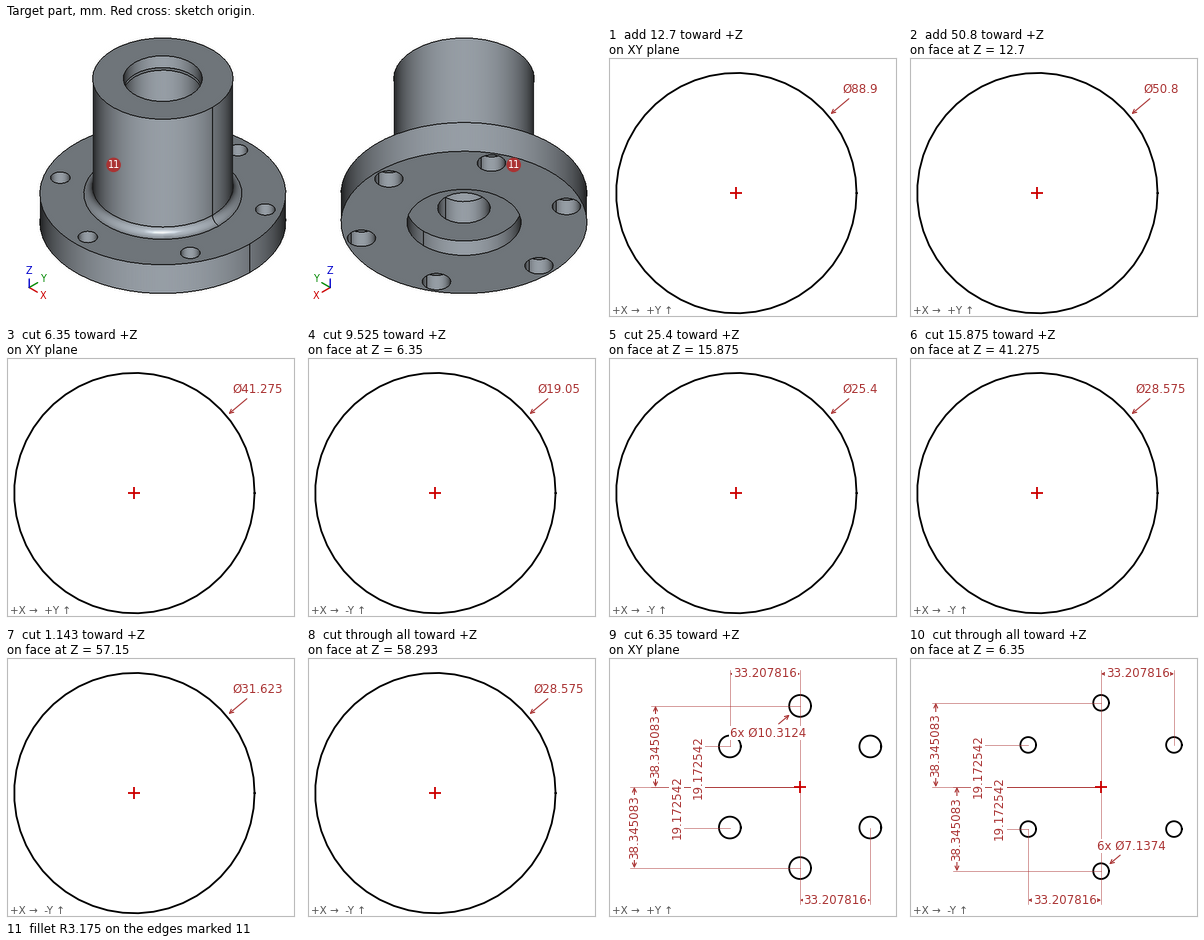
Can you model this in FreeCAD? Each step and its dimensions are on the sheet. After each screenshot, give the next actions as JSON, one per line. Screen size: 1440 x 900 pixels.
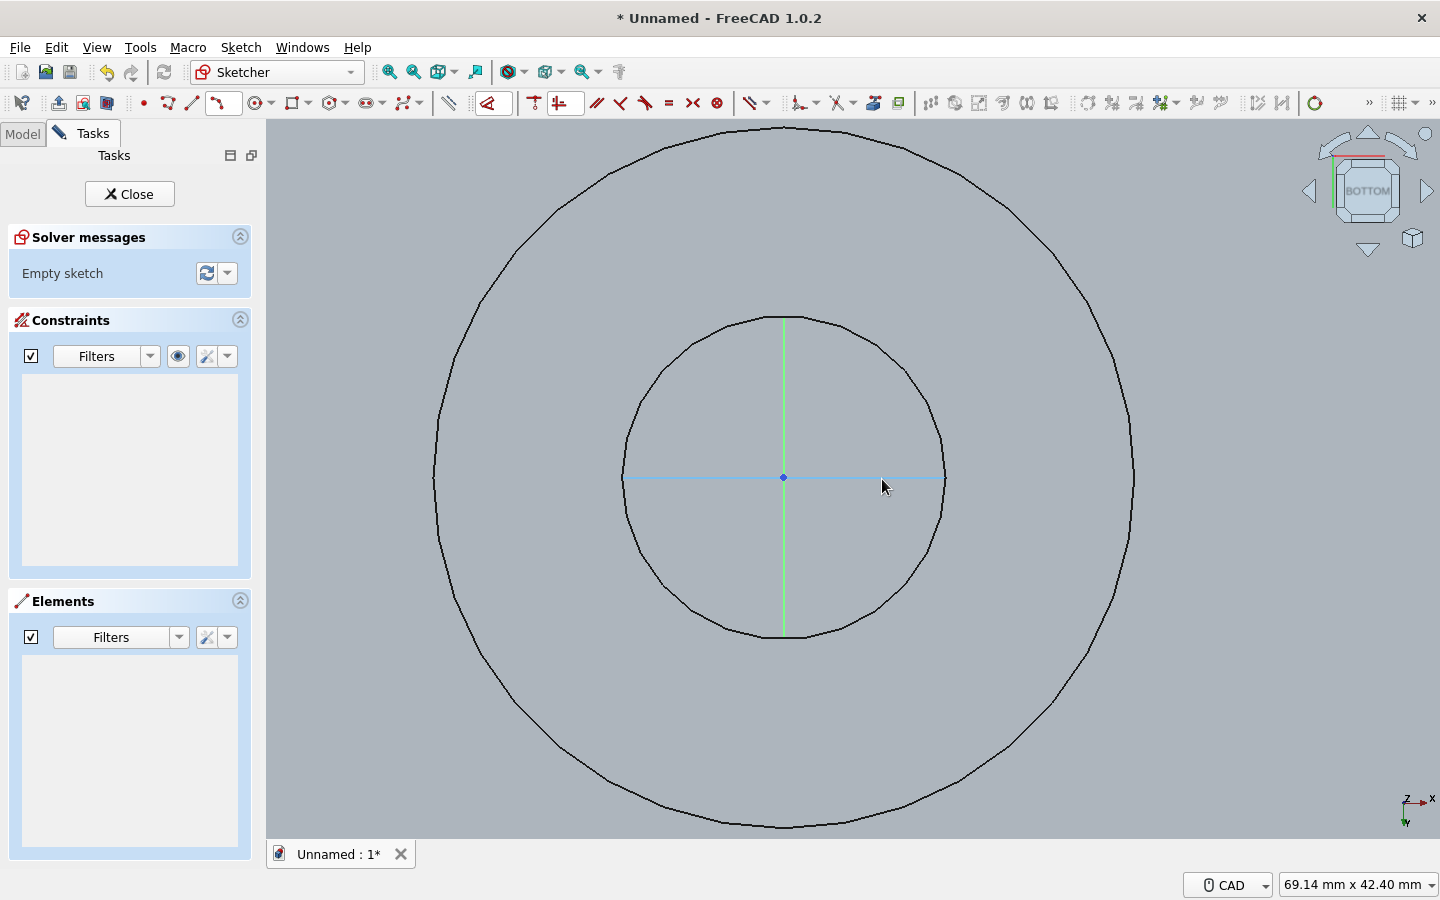
{"action": "left_click", "coordinate": [256, 104]}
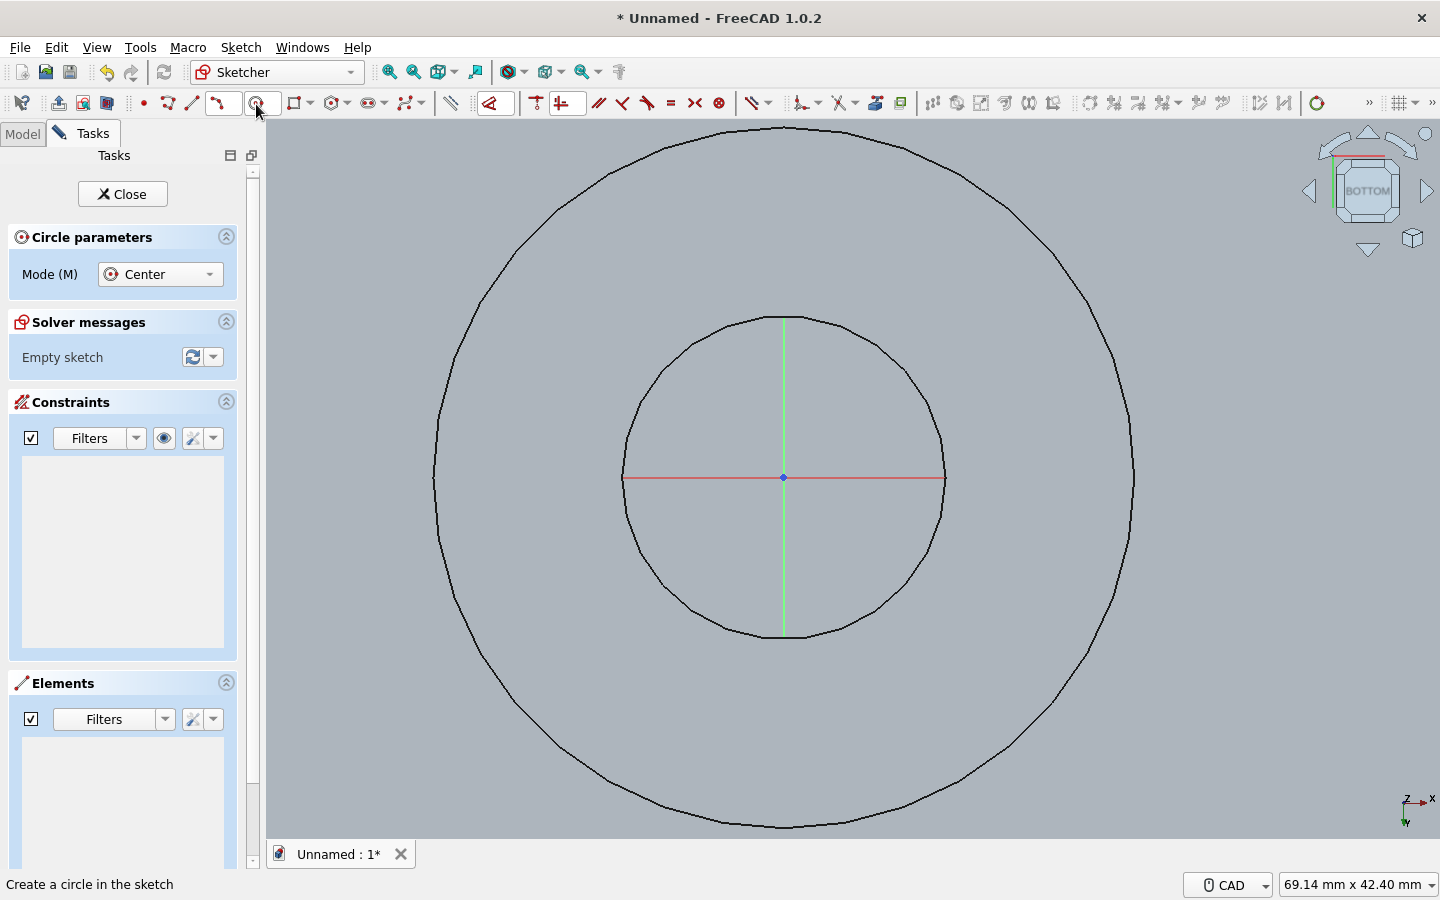
{"action": "left_click", "coordinate": [784, 478]}
{"action": "mouse_move", "coordinate": [936, 325]}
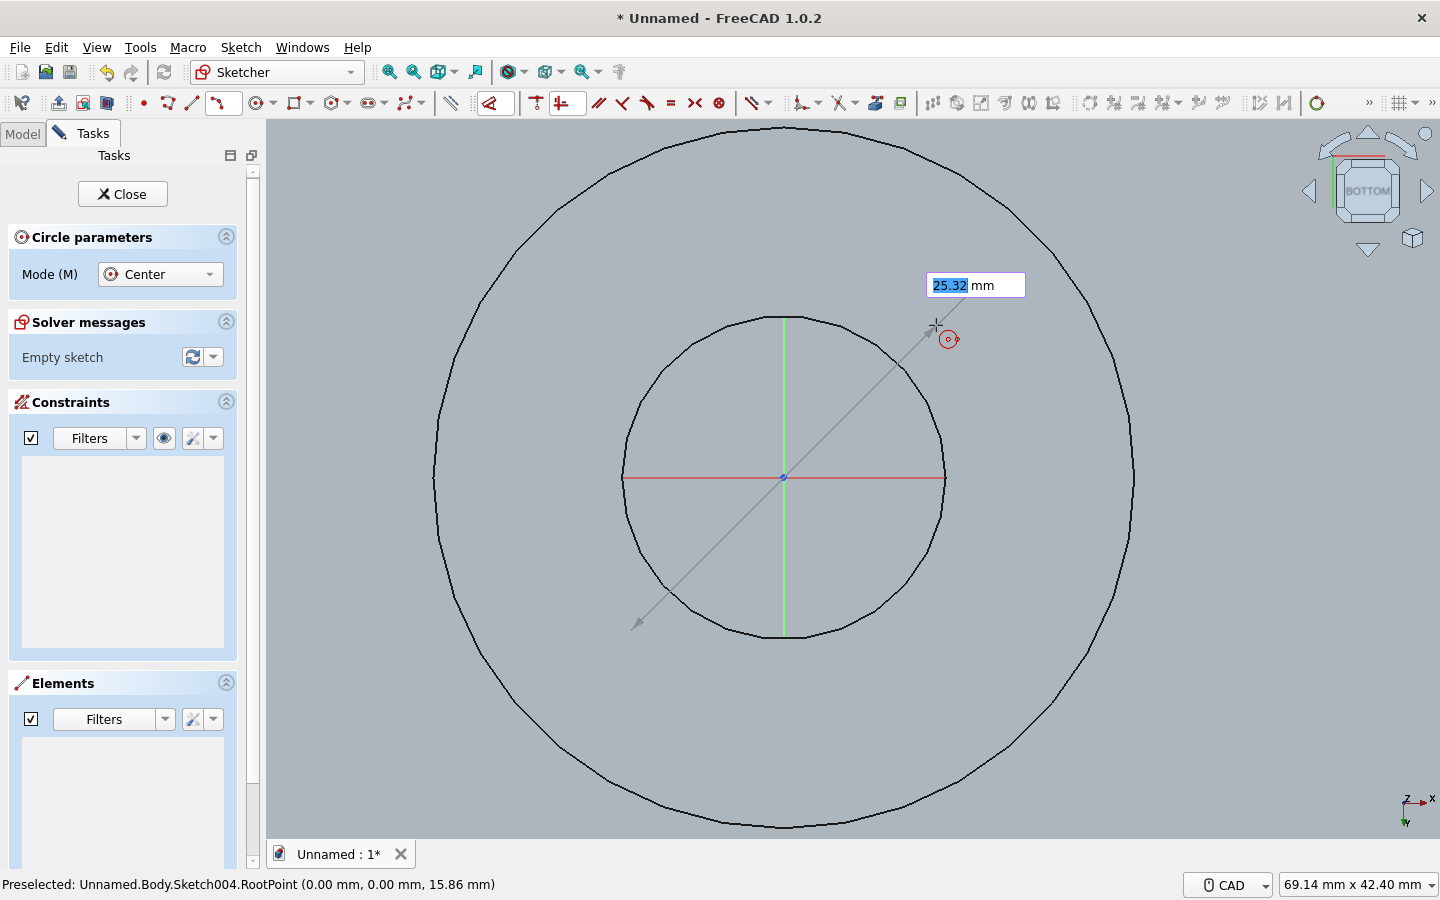
{"action": "type", "text": "25.4"}
{"action": "key", "text": "Return"}
{"action": "key", "text": "Escape"}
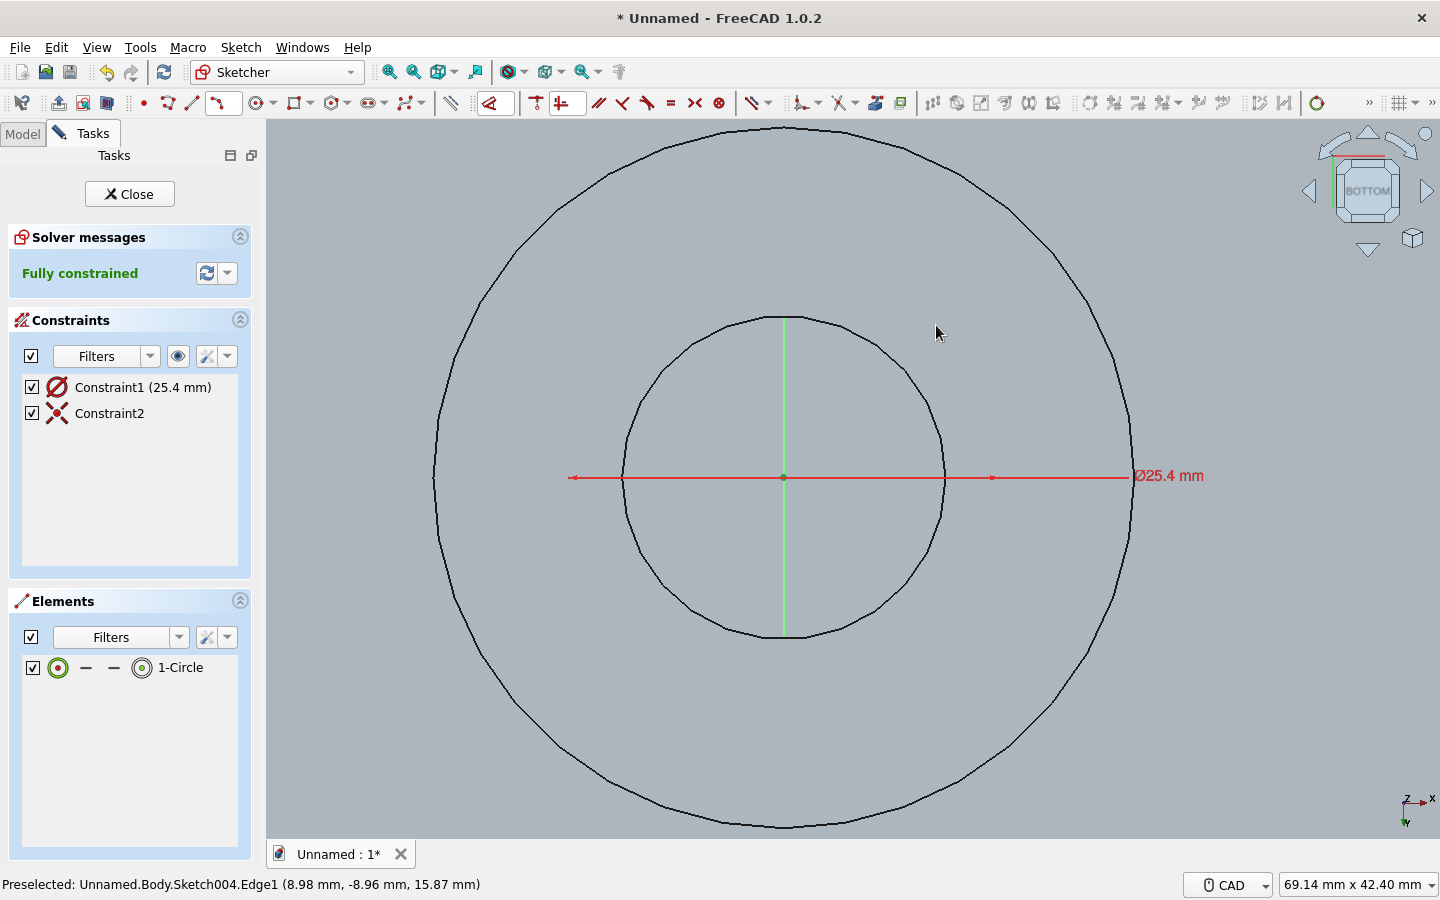
{"action": "left_click", "coordinate": [130, 194]}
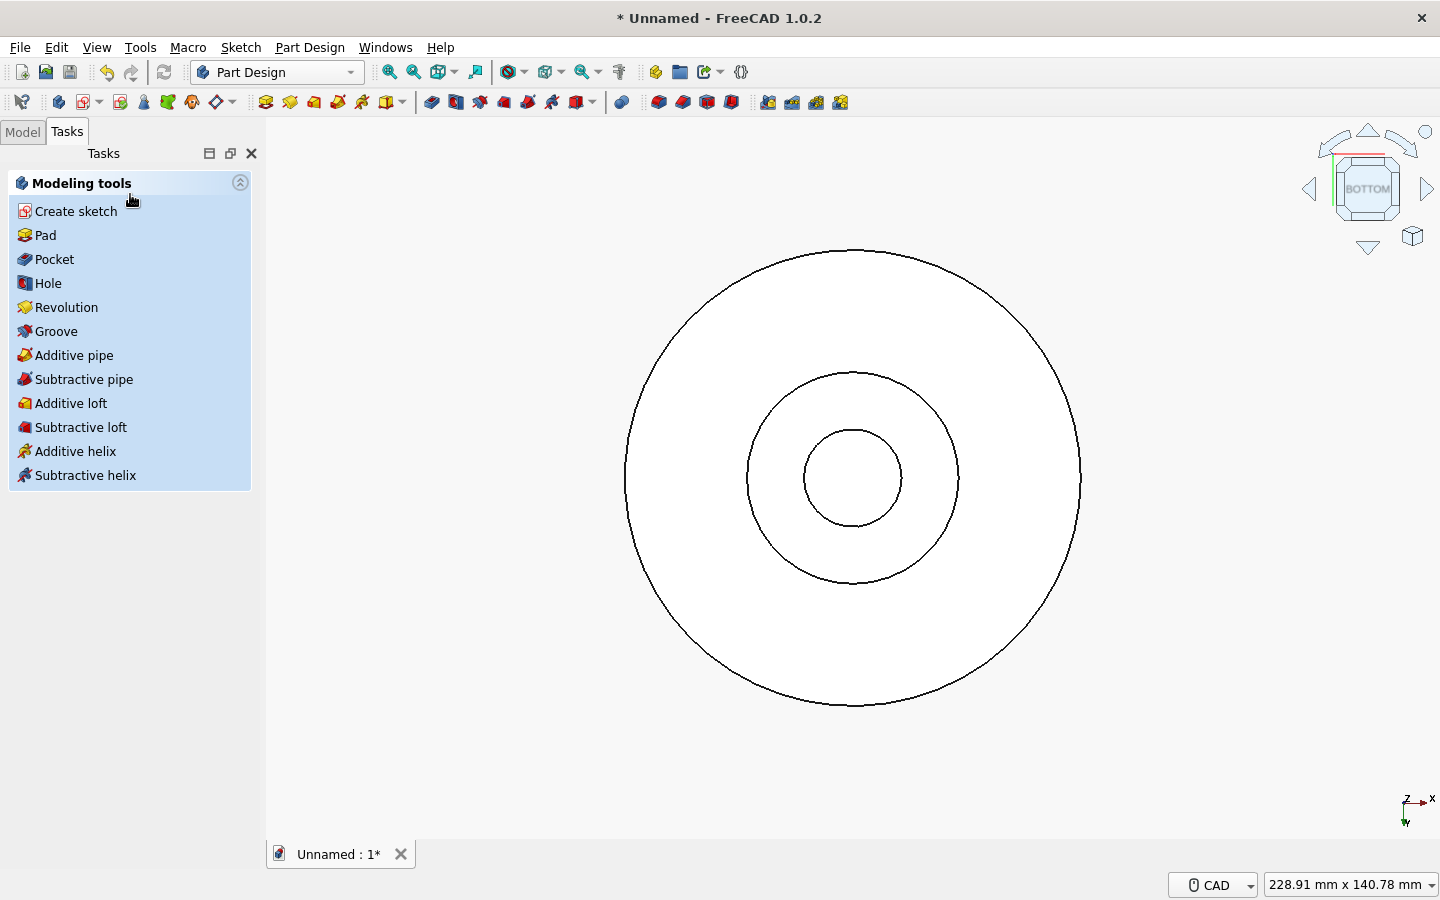
{"action": "left_click", "coordinate": [432, 102]}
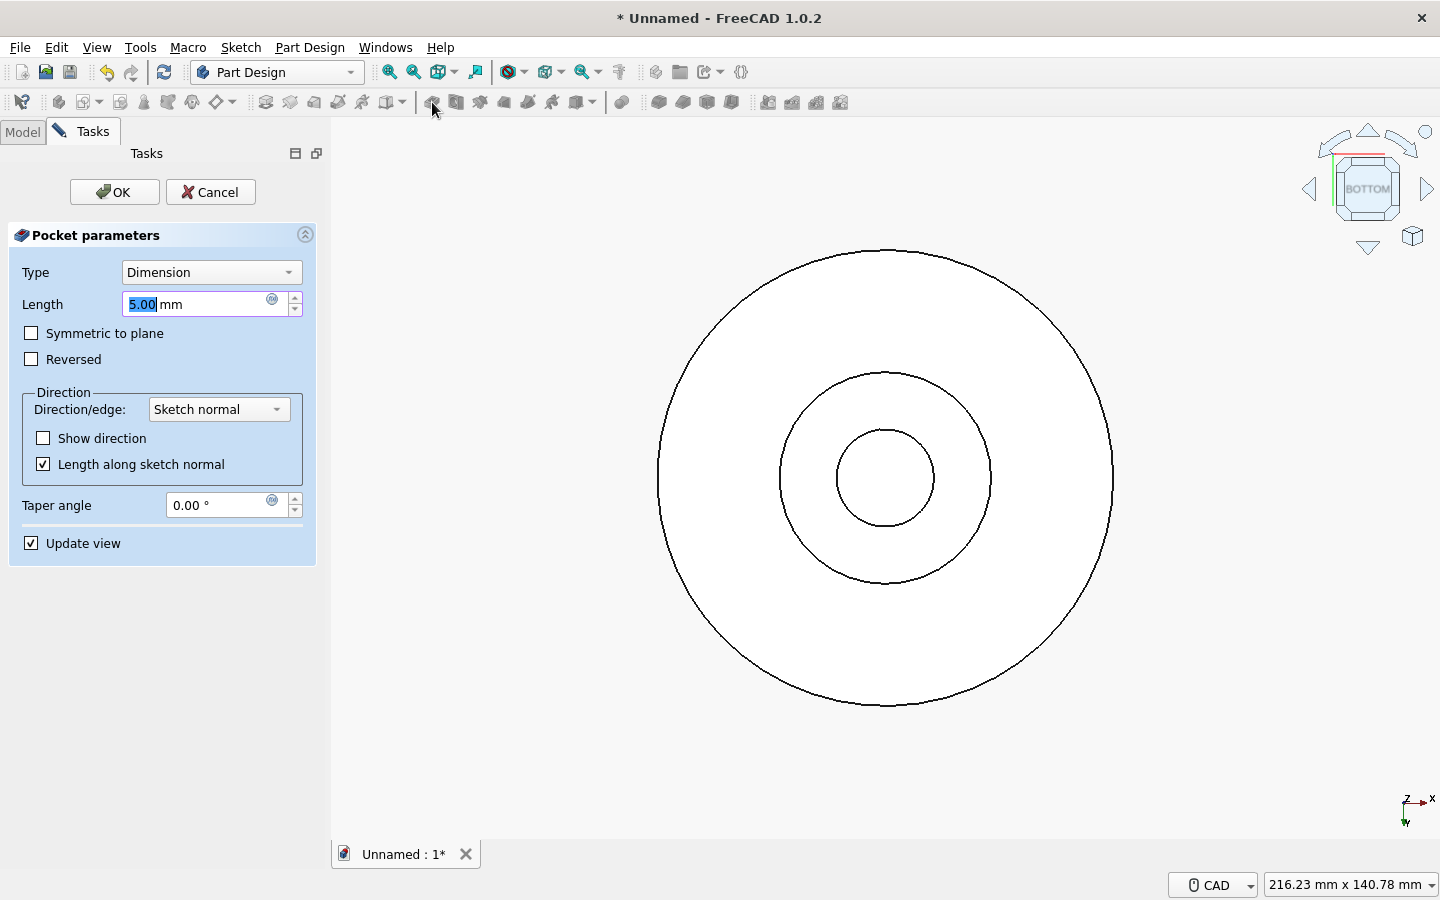
{"action": "type", "text": "25.4"}
{"action": "key", "text": "Tab"}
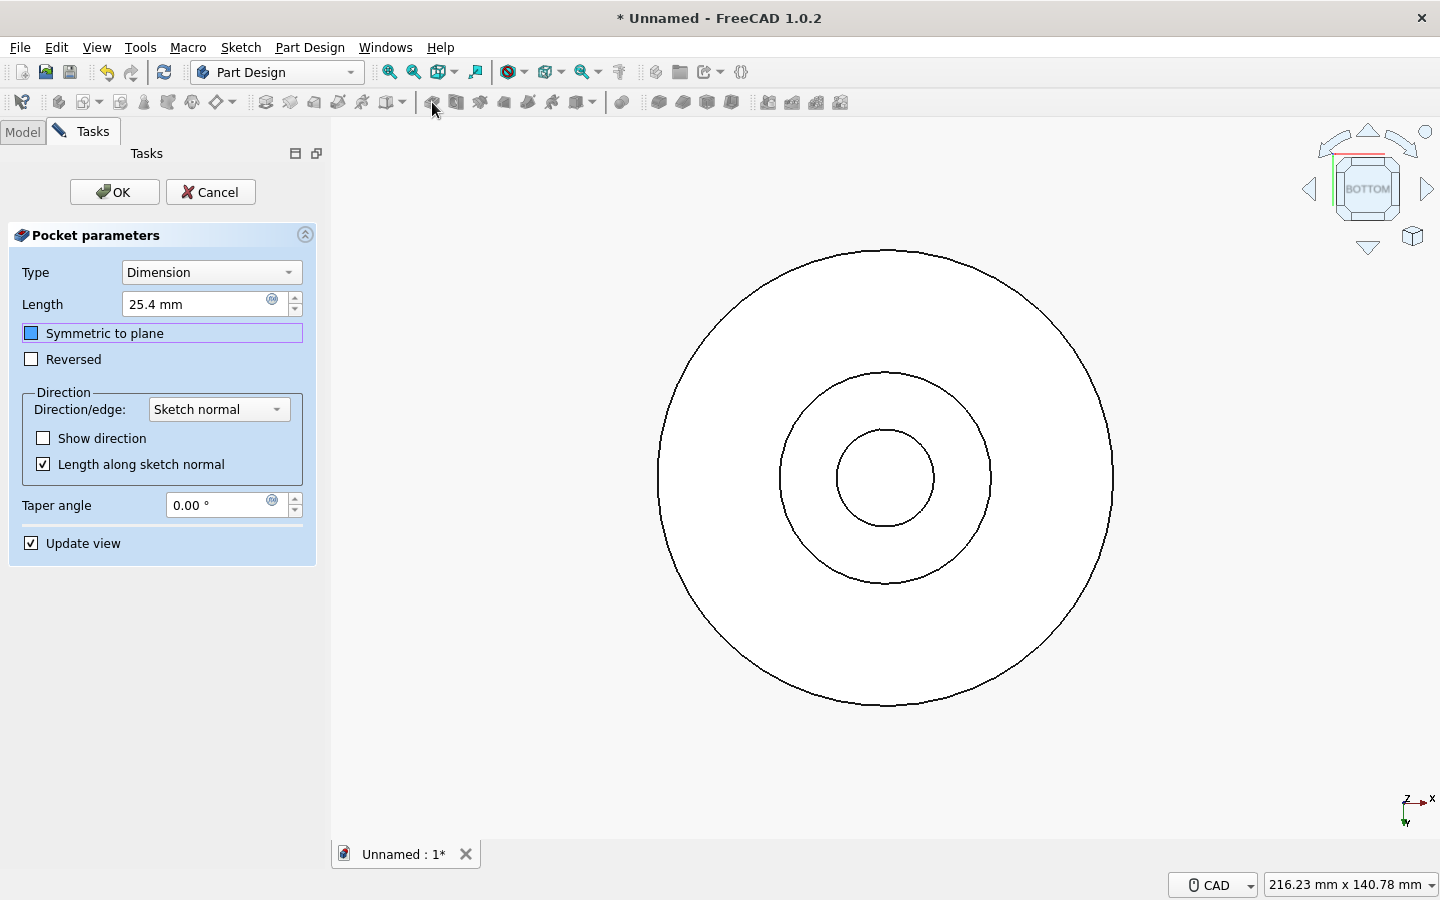
{"action": "left_click", "coordinate": [115, 192]}